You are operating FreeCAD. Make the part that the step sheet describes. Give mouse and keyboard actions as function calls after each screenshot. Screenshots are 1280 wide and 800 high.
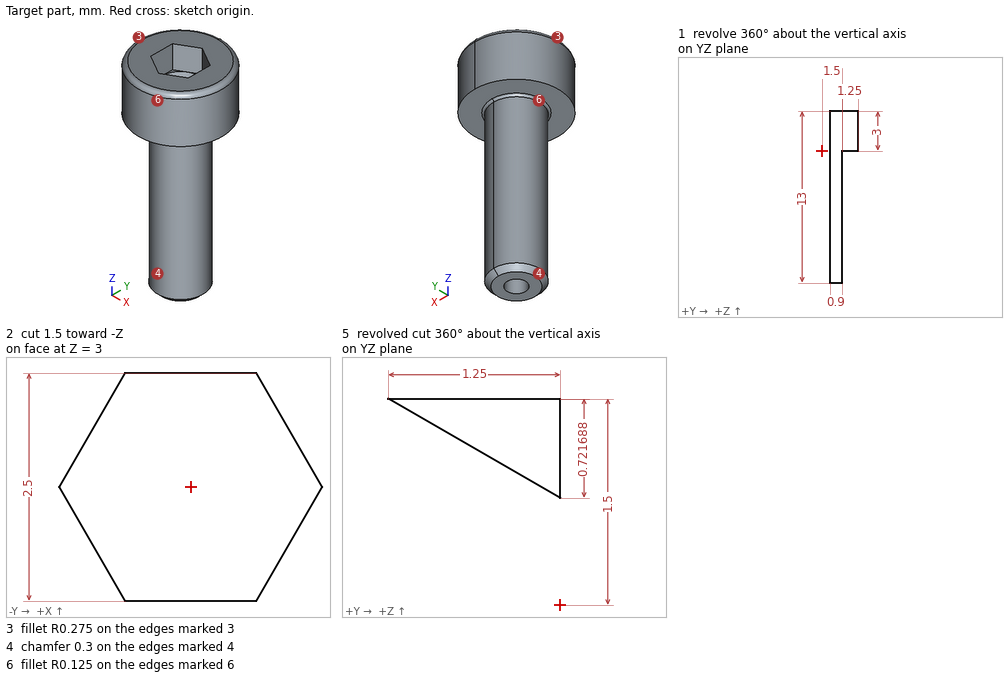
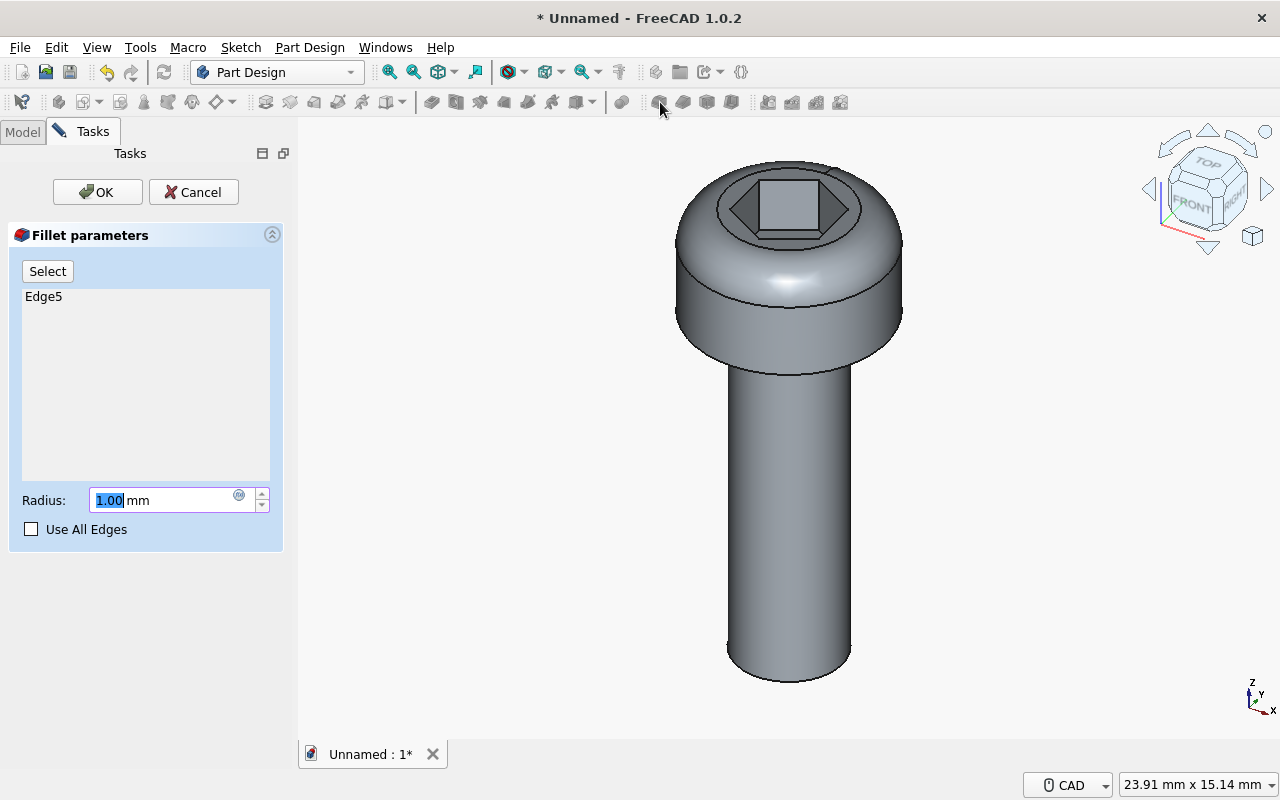
text(0.275)
key(Tab)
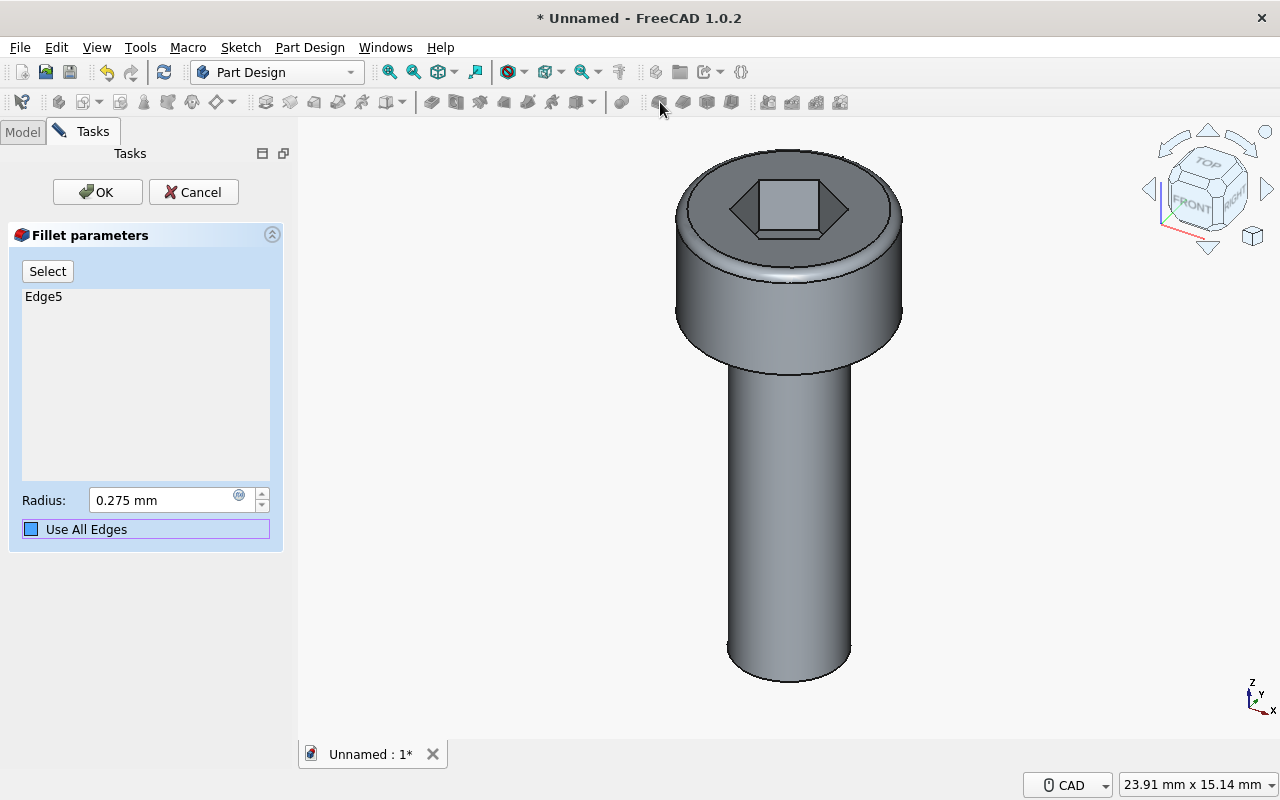
click(98, 192)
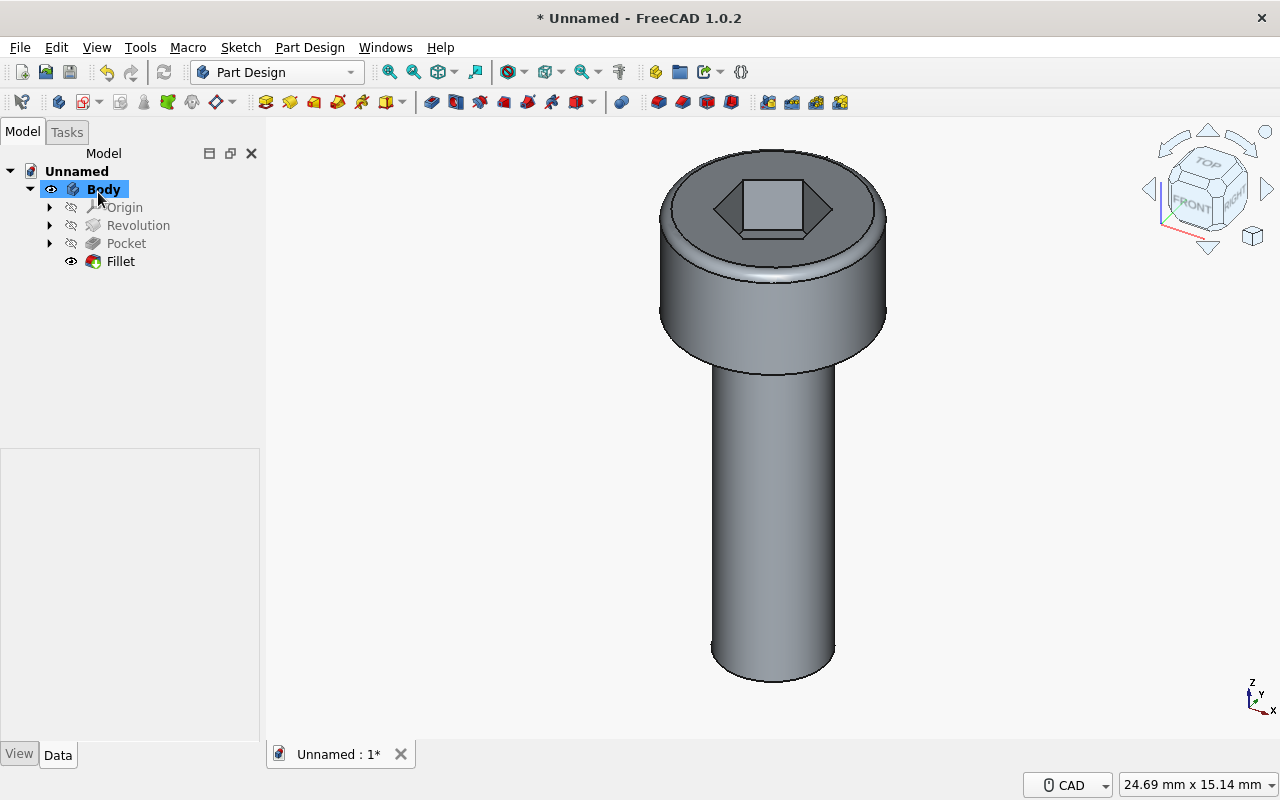
key(0)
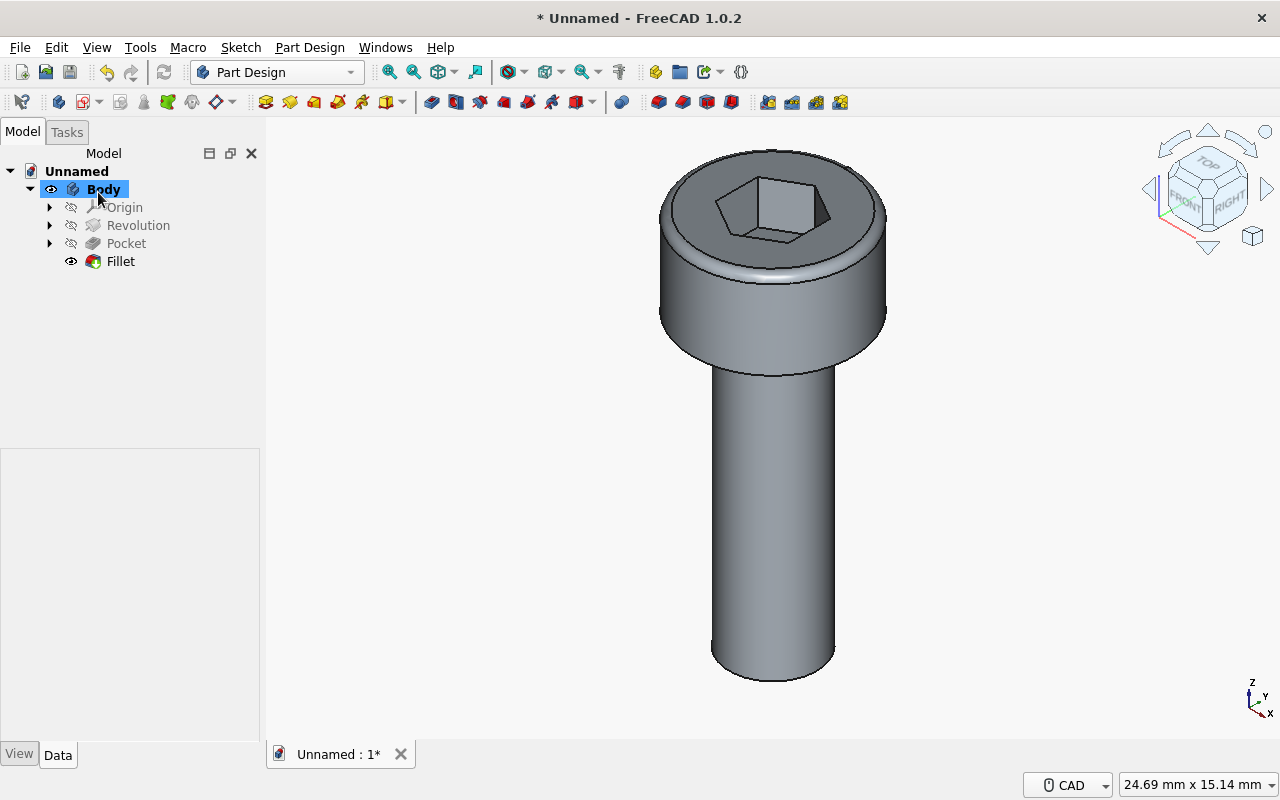
key(2)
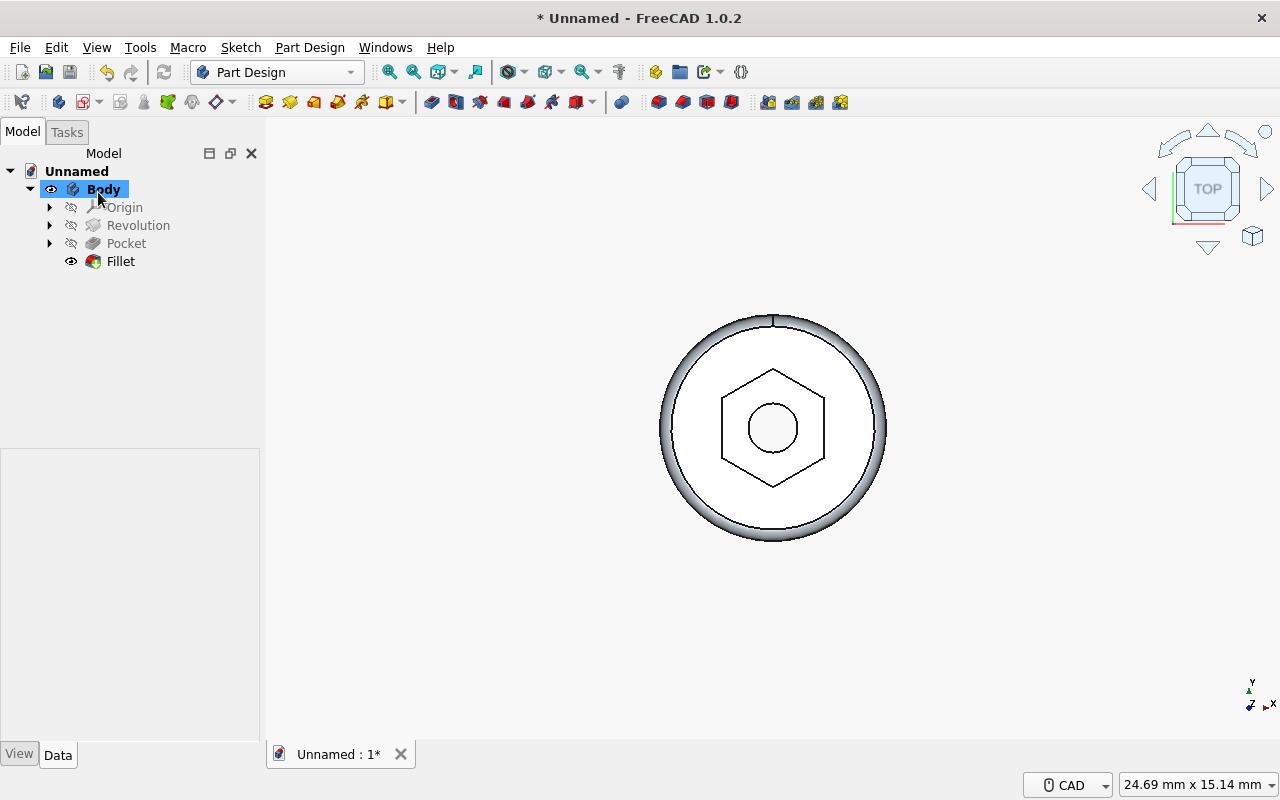
click(390, 72)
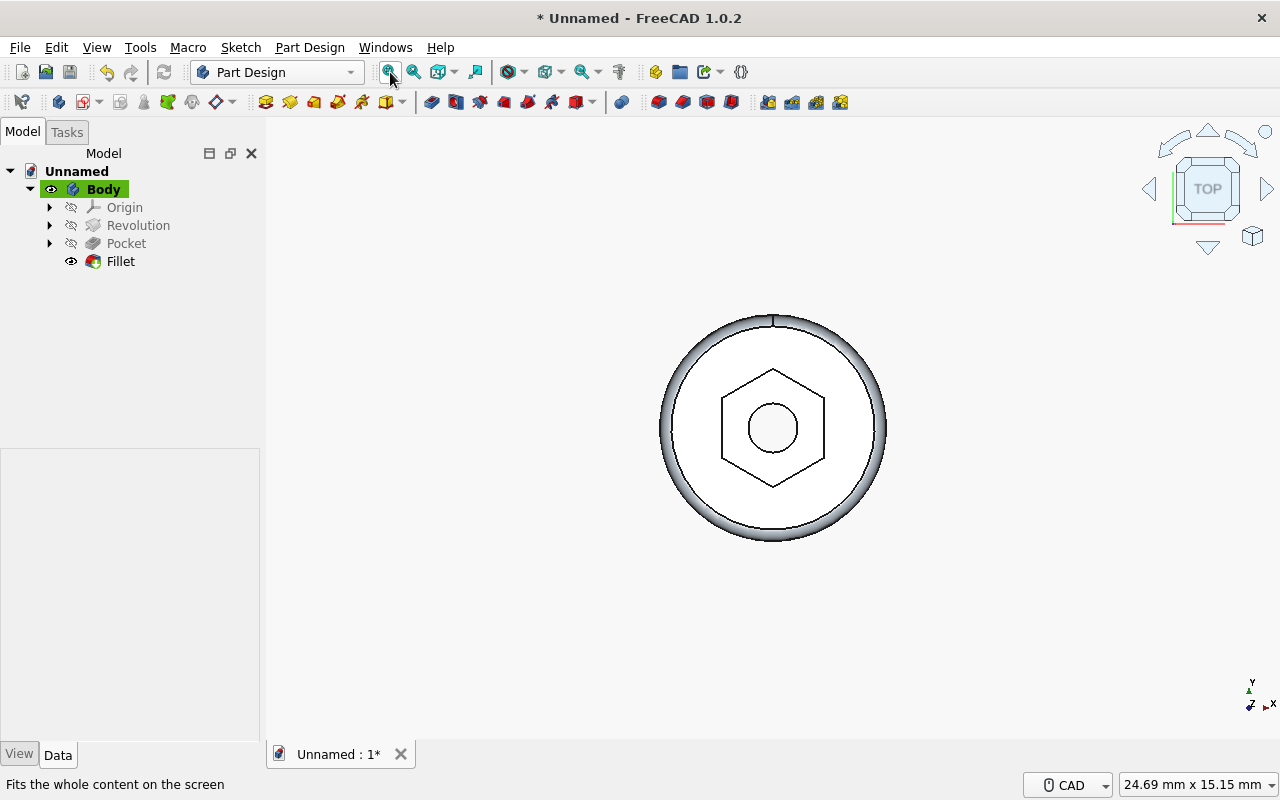
key(1)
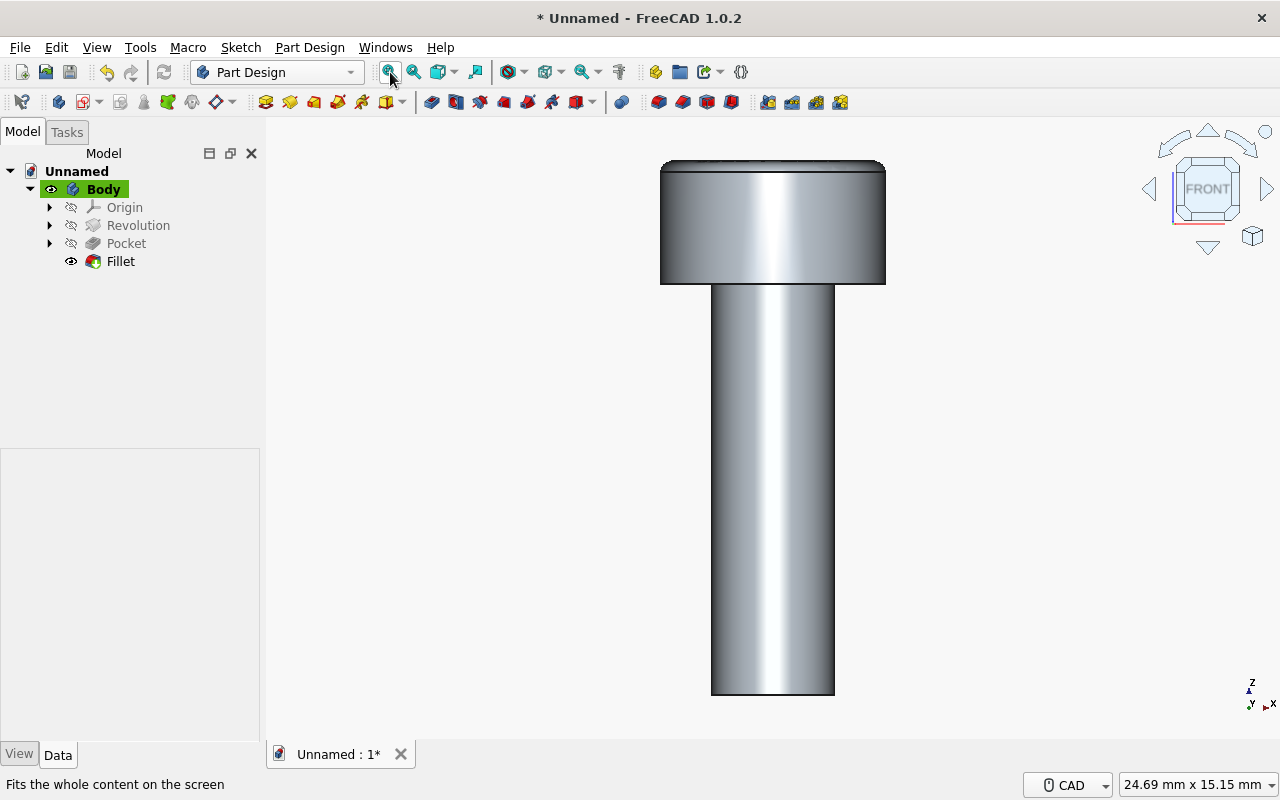
click(773, 694)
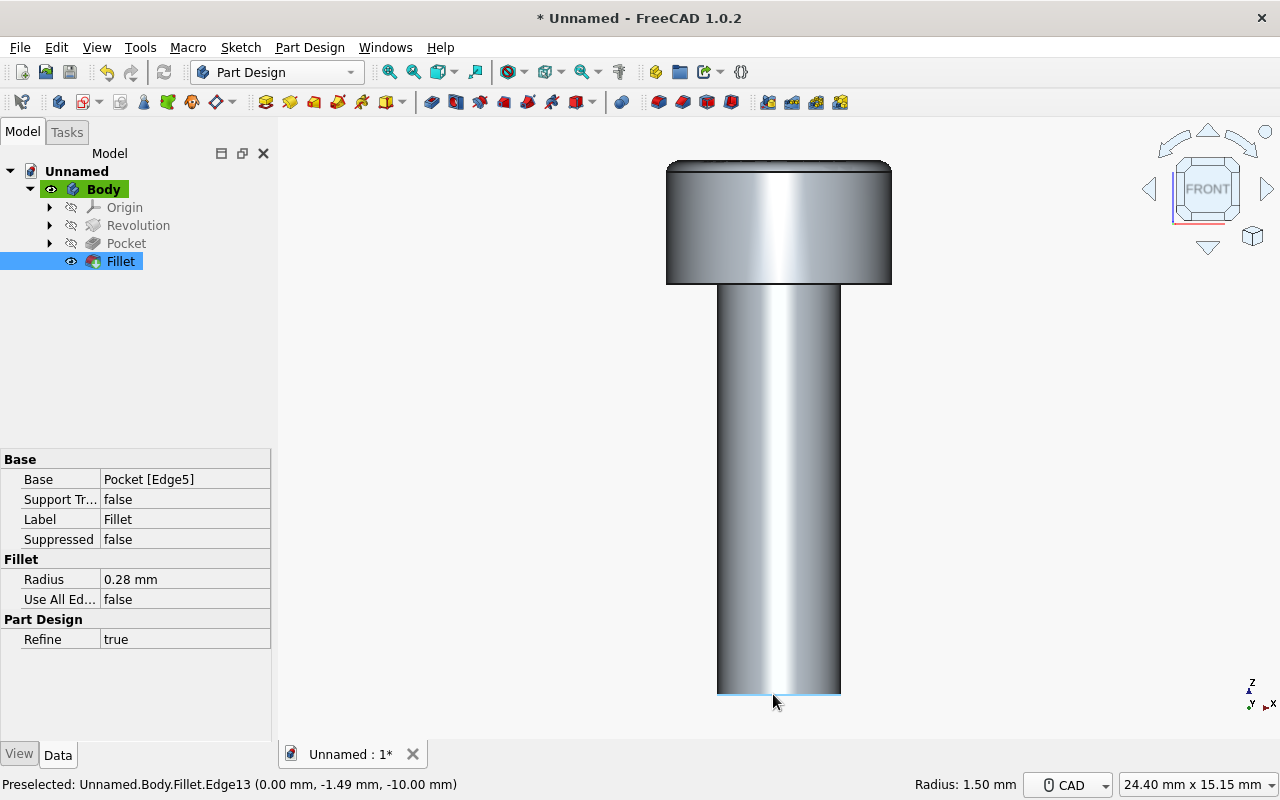
click(684, 102)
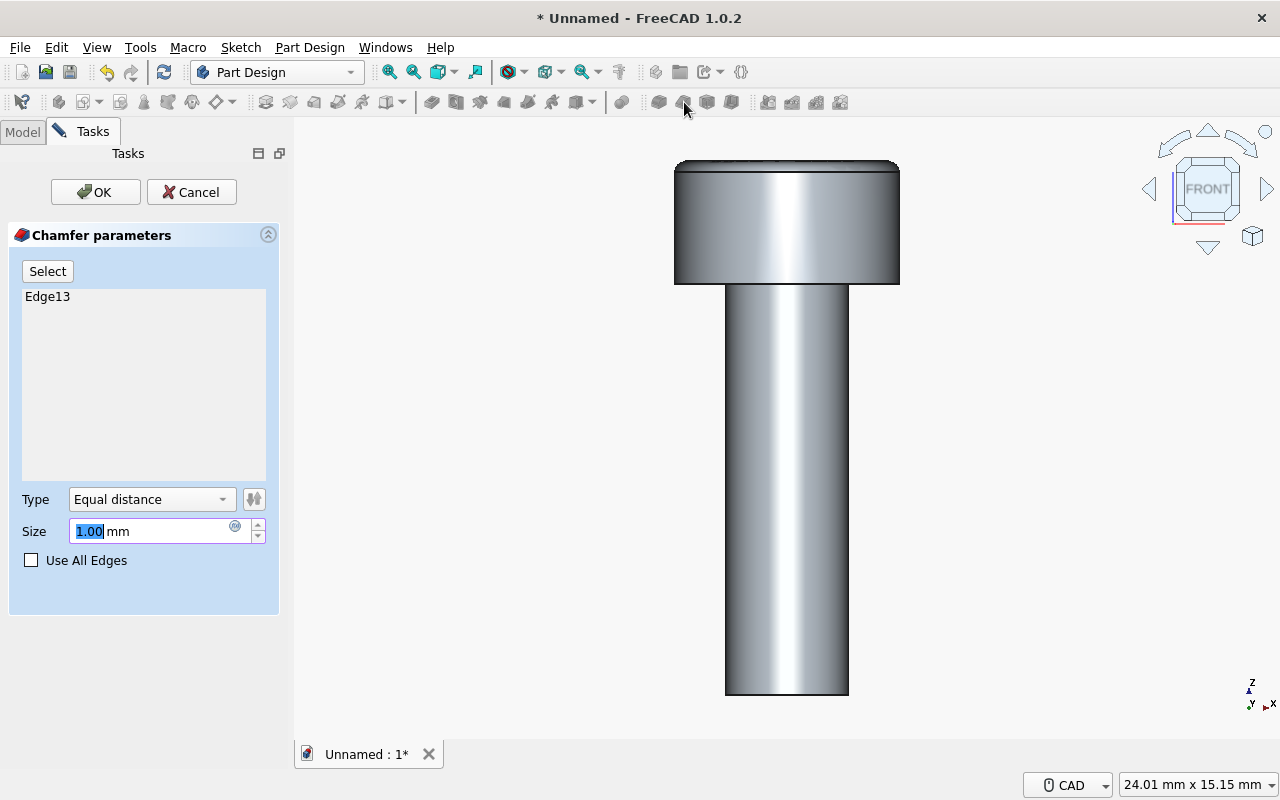
text(0.3)
key(Tab)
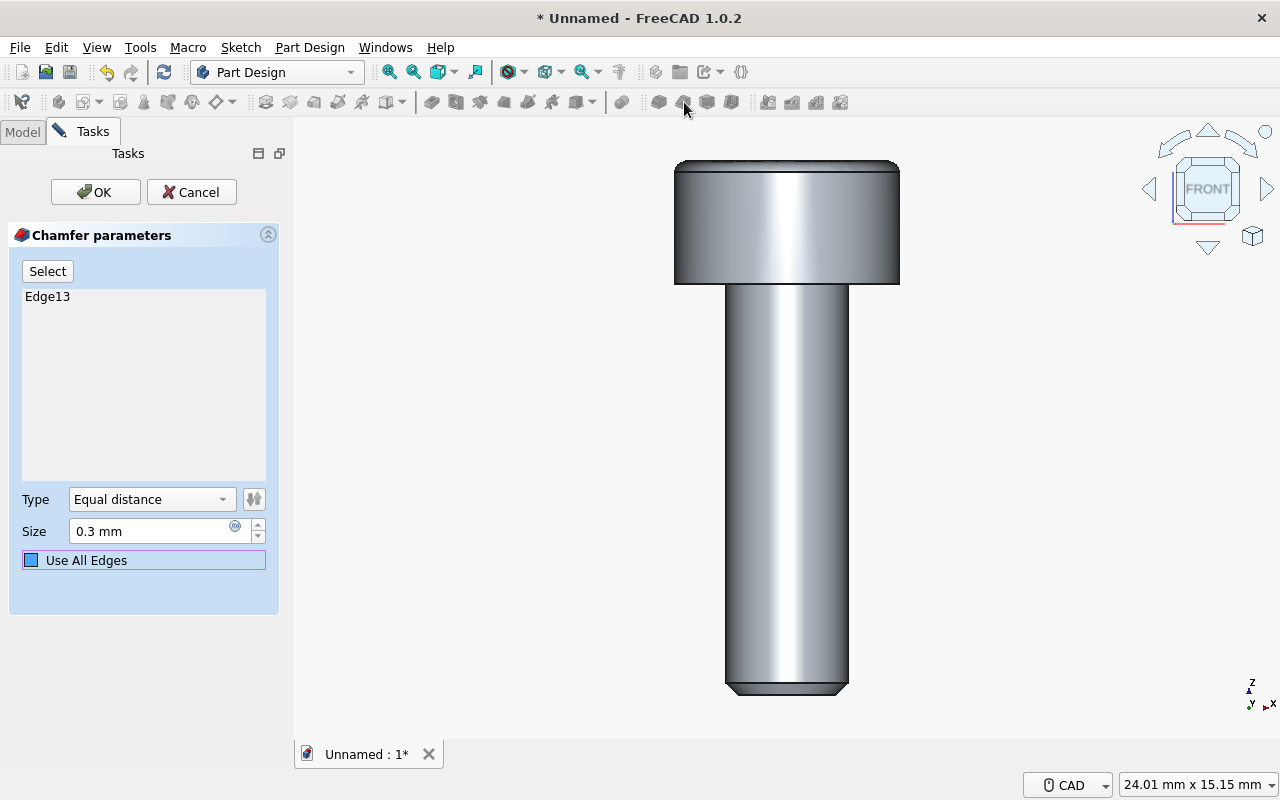
click(96, 192)